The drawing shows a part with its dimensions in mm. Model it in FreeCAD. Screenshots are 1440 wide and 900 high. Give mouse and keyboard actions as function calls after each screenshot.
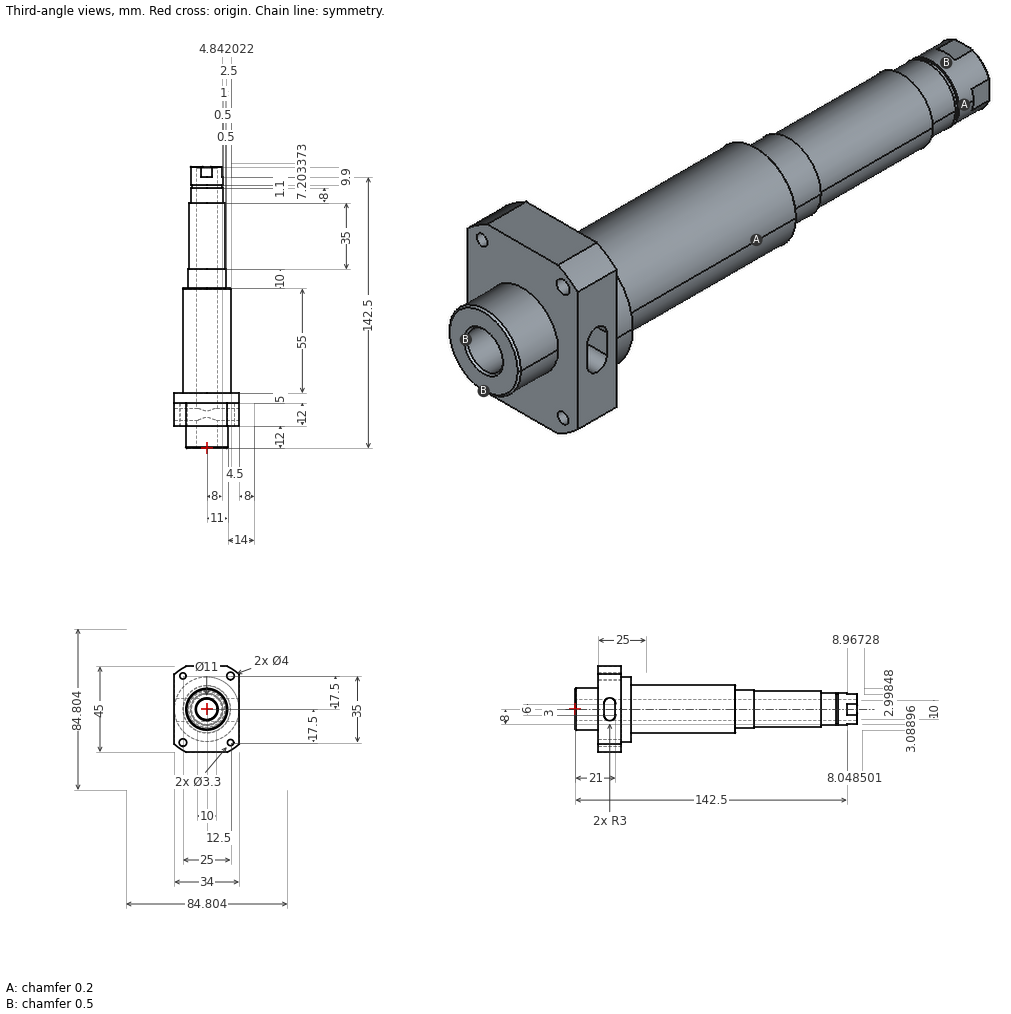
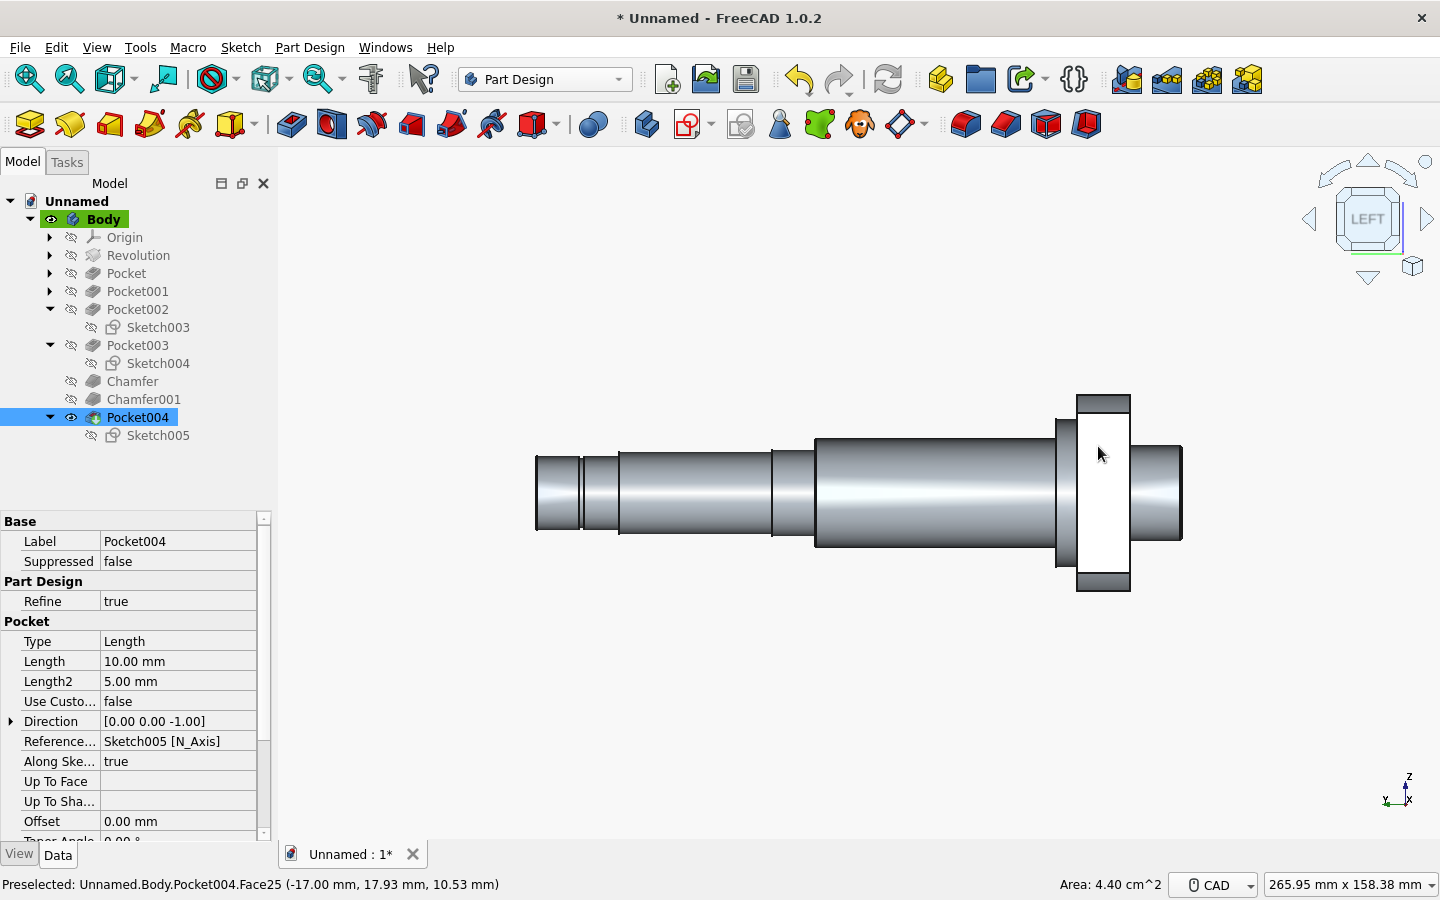
click(688, 124)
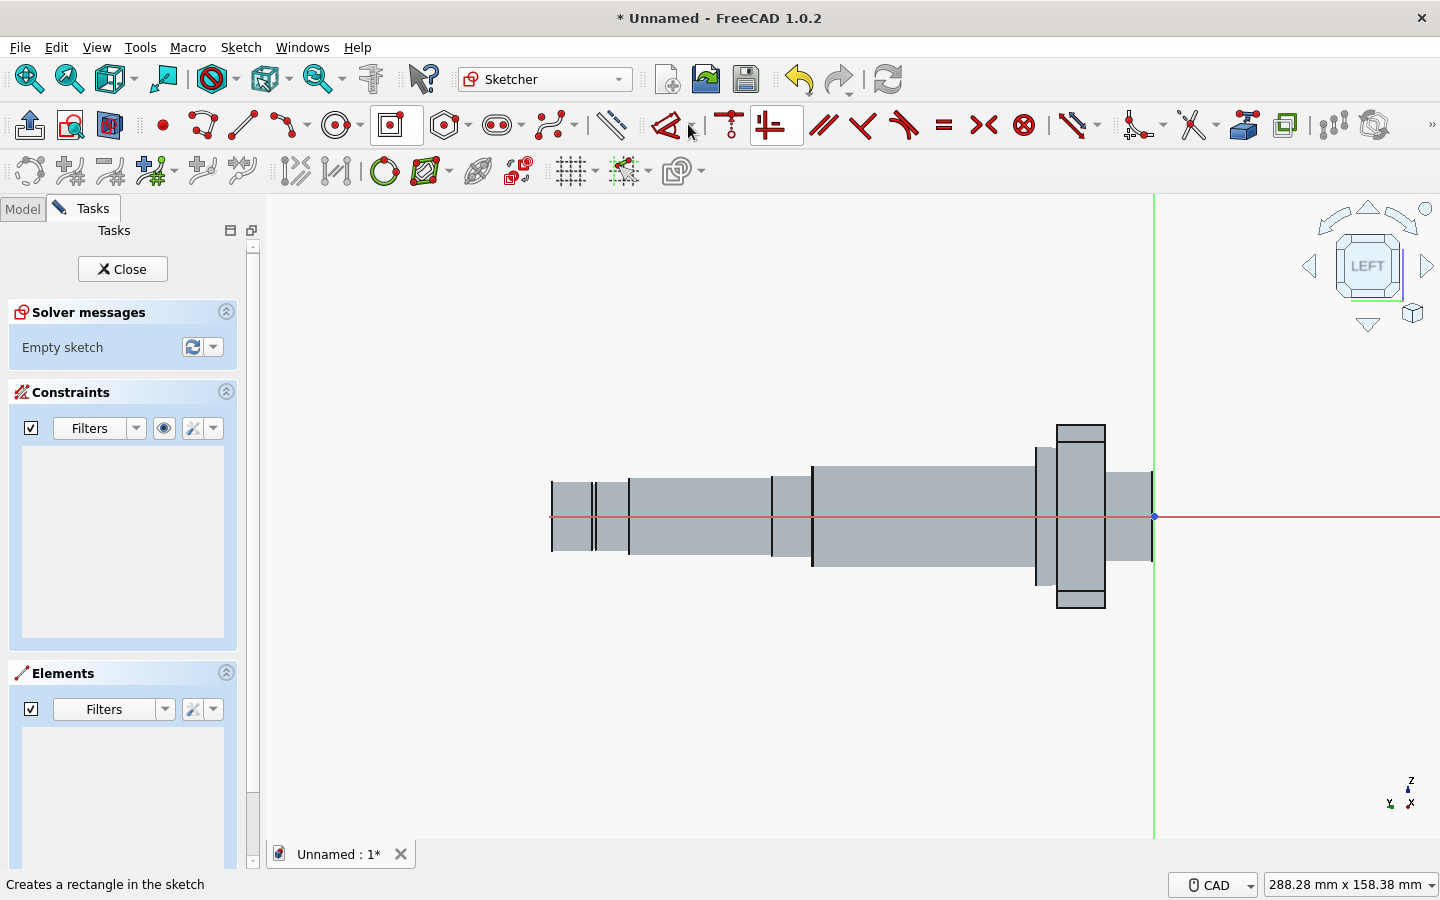
scroll(1163, 516, up, 10)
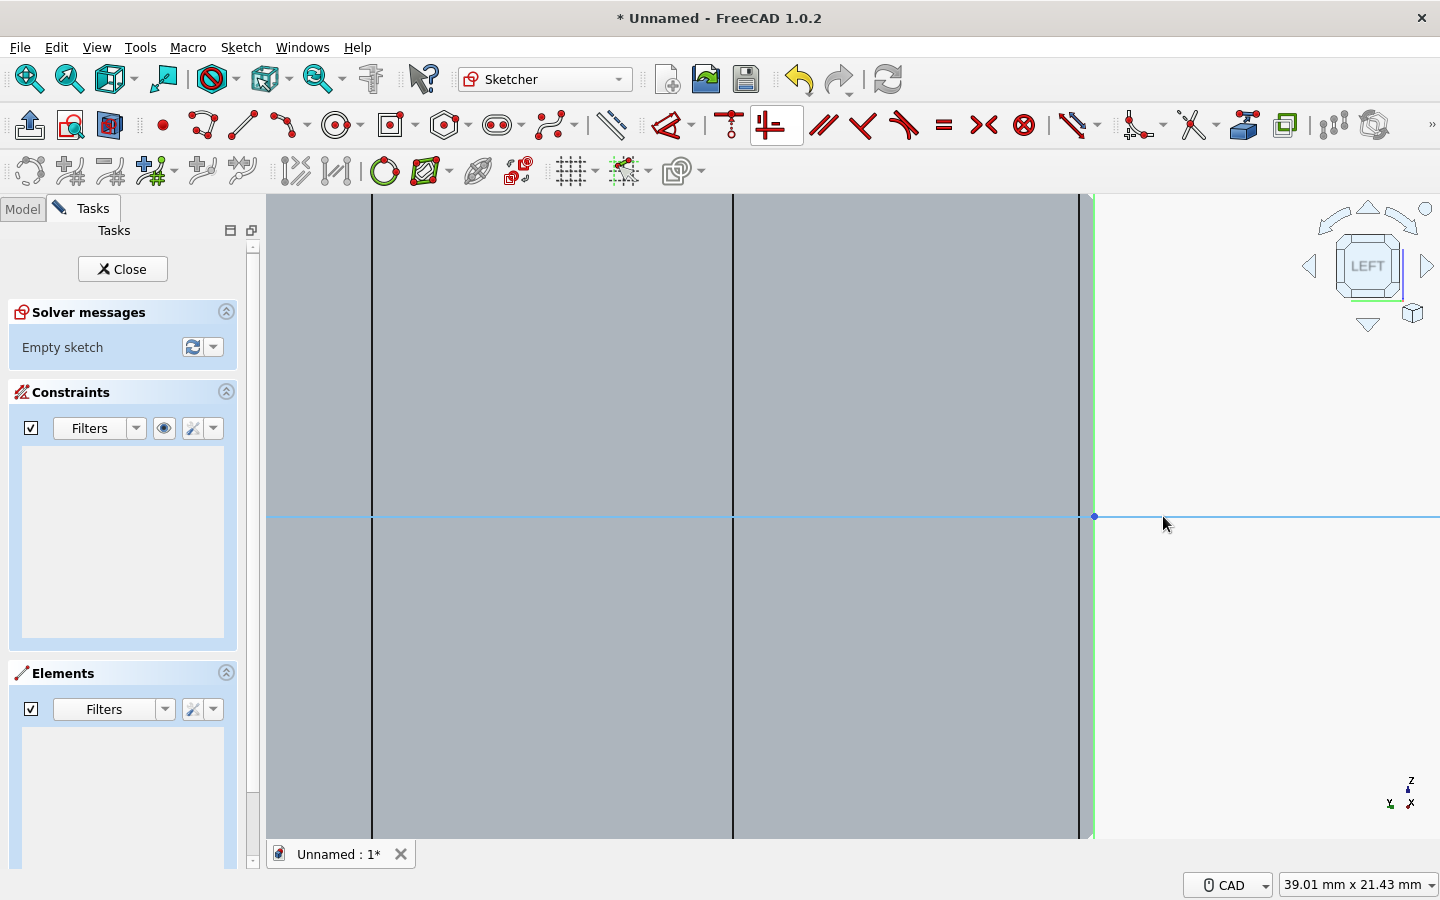
key(g)
key(s)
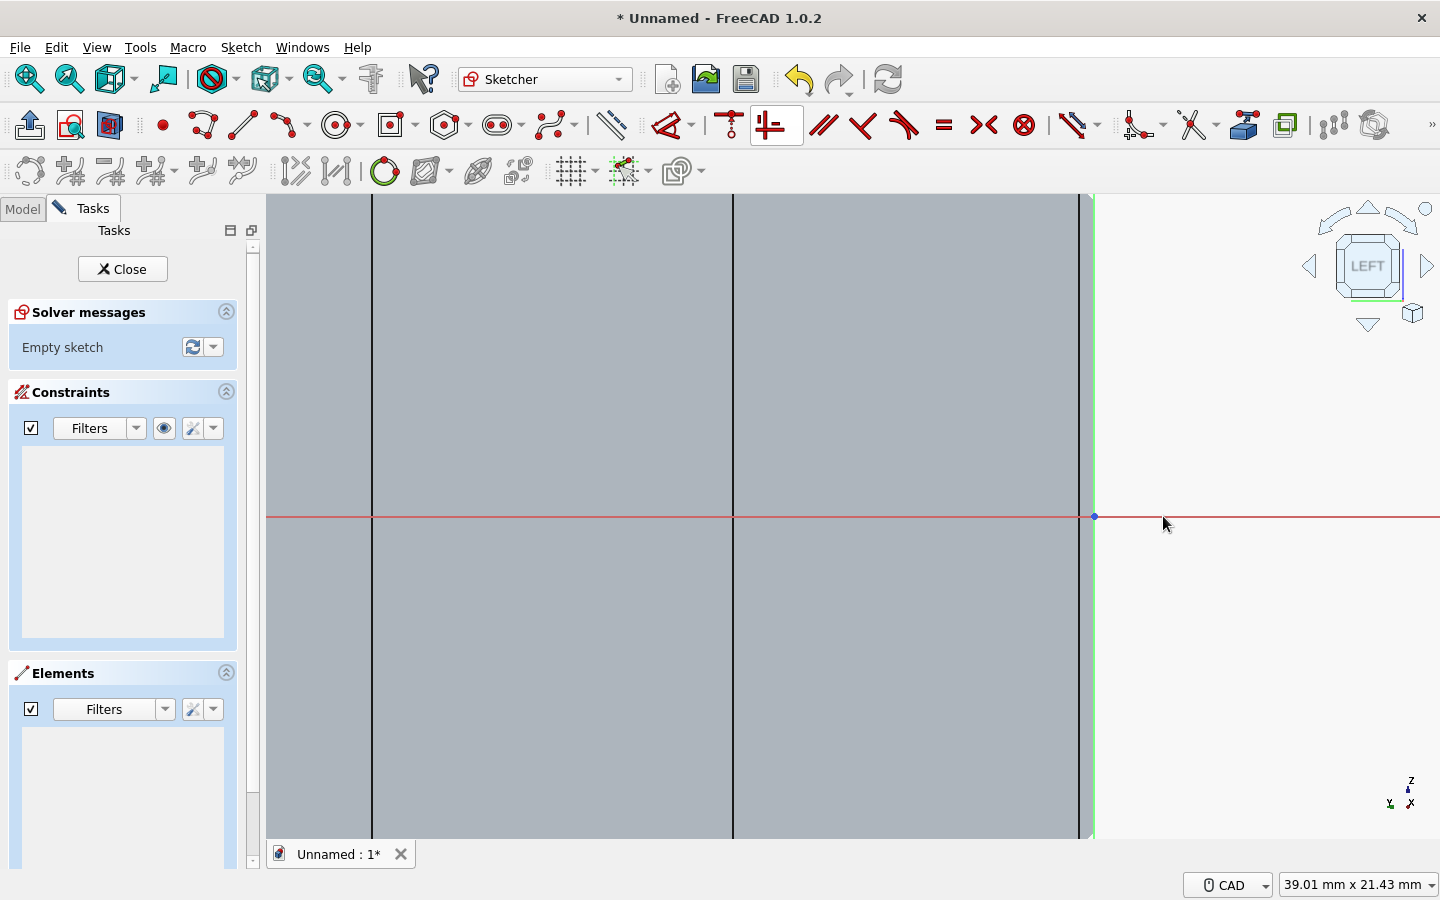
click(553, 607)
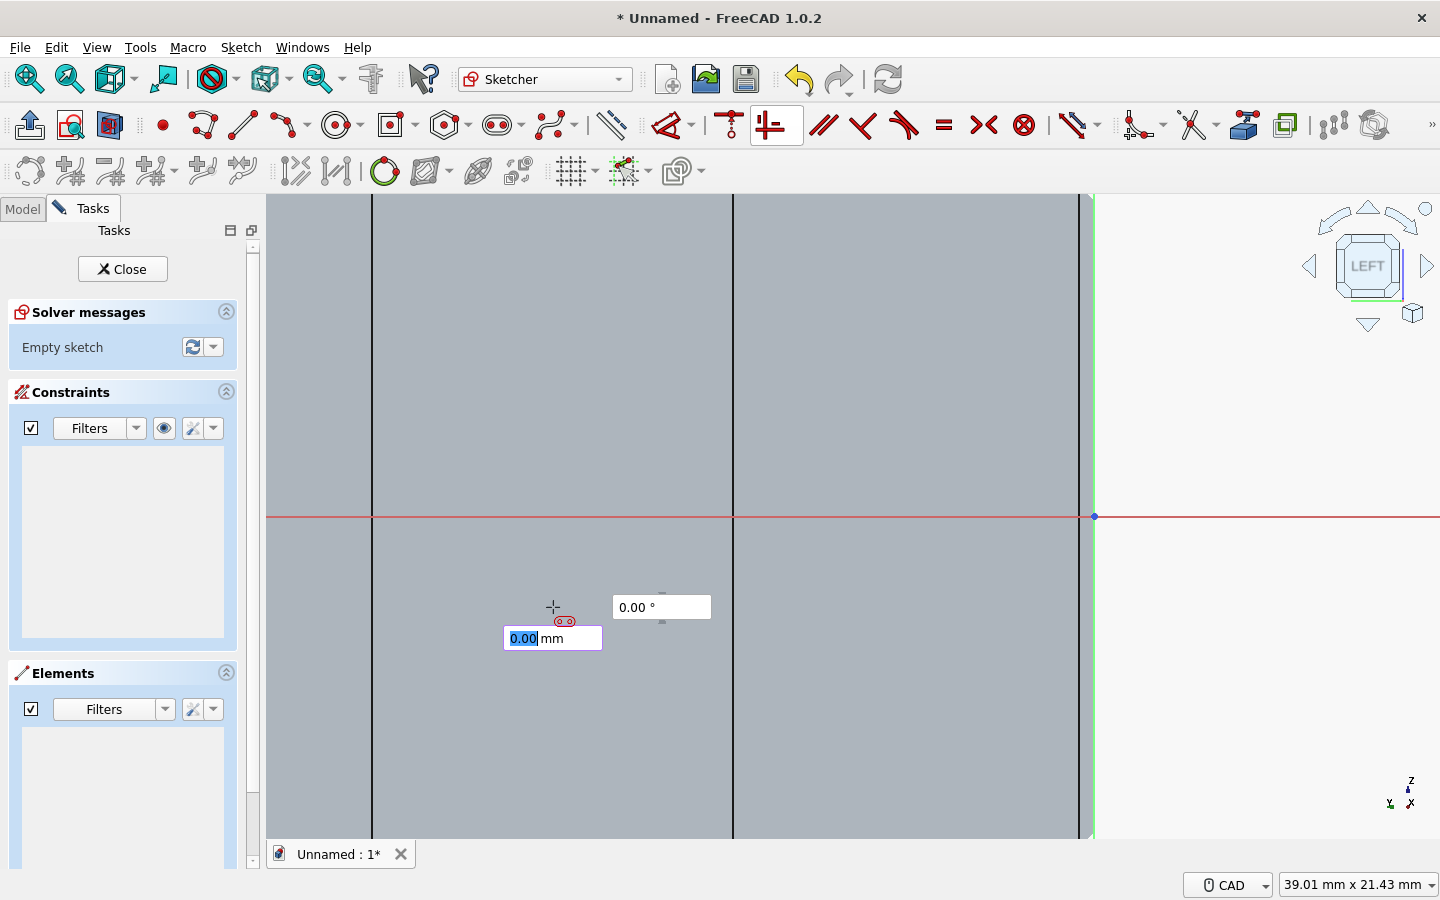
click(553, 426)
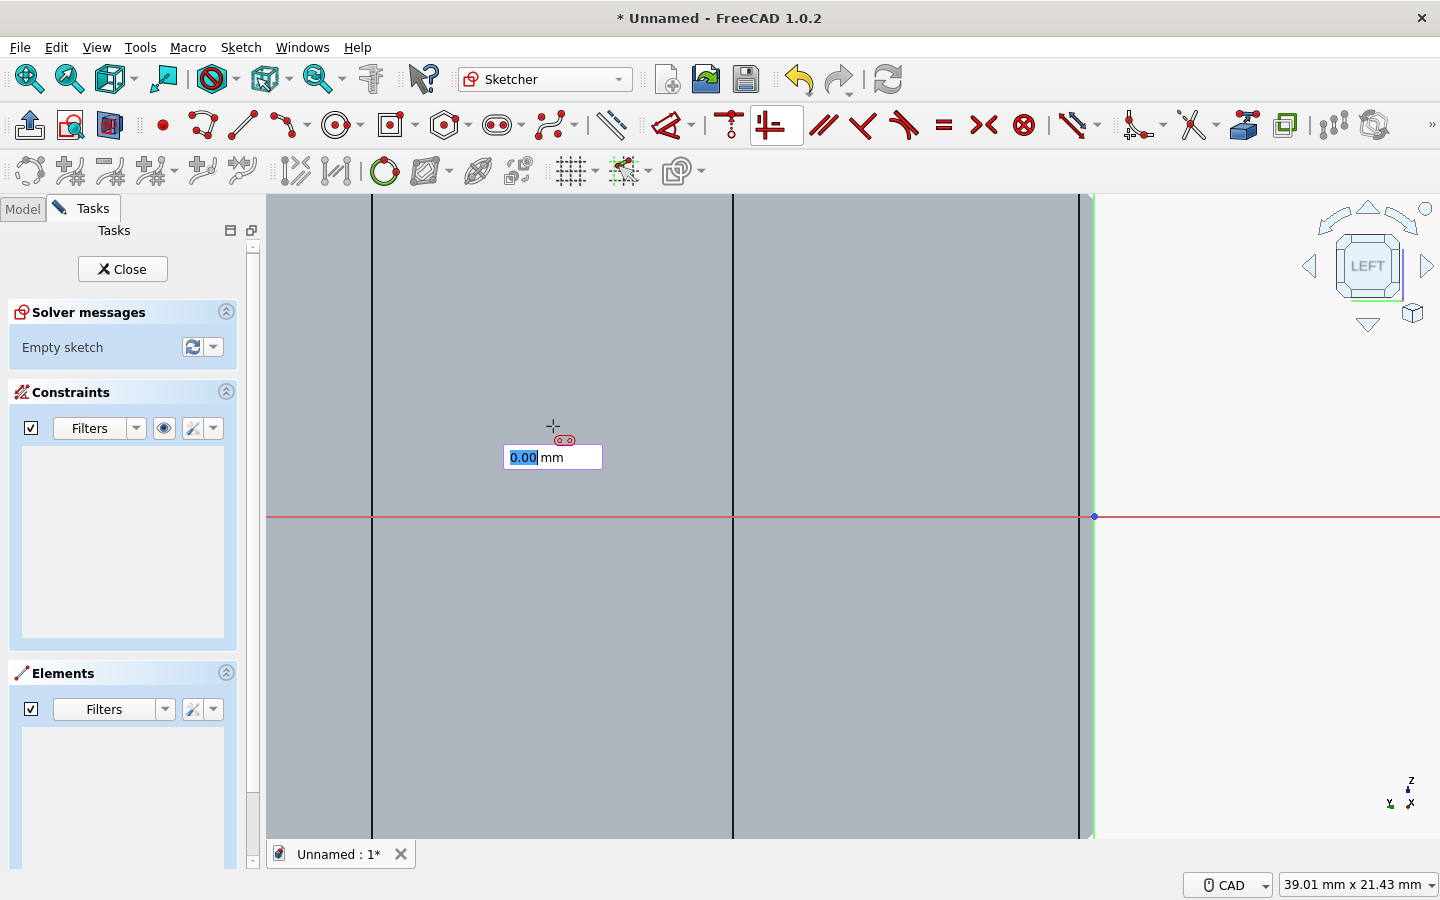
click(462, 489)
key(Escape)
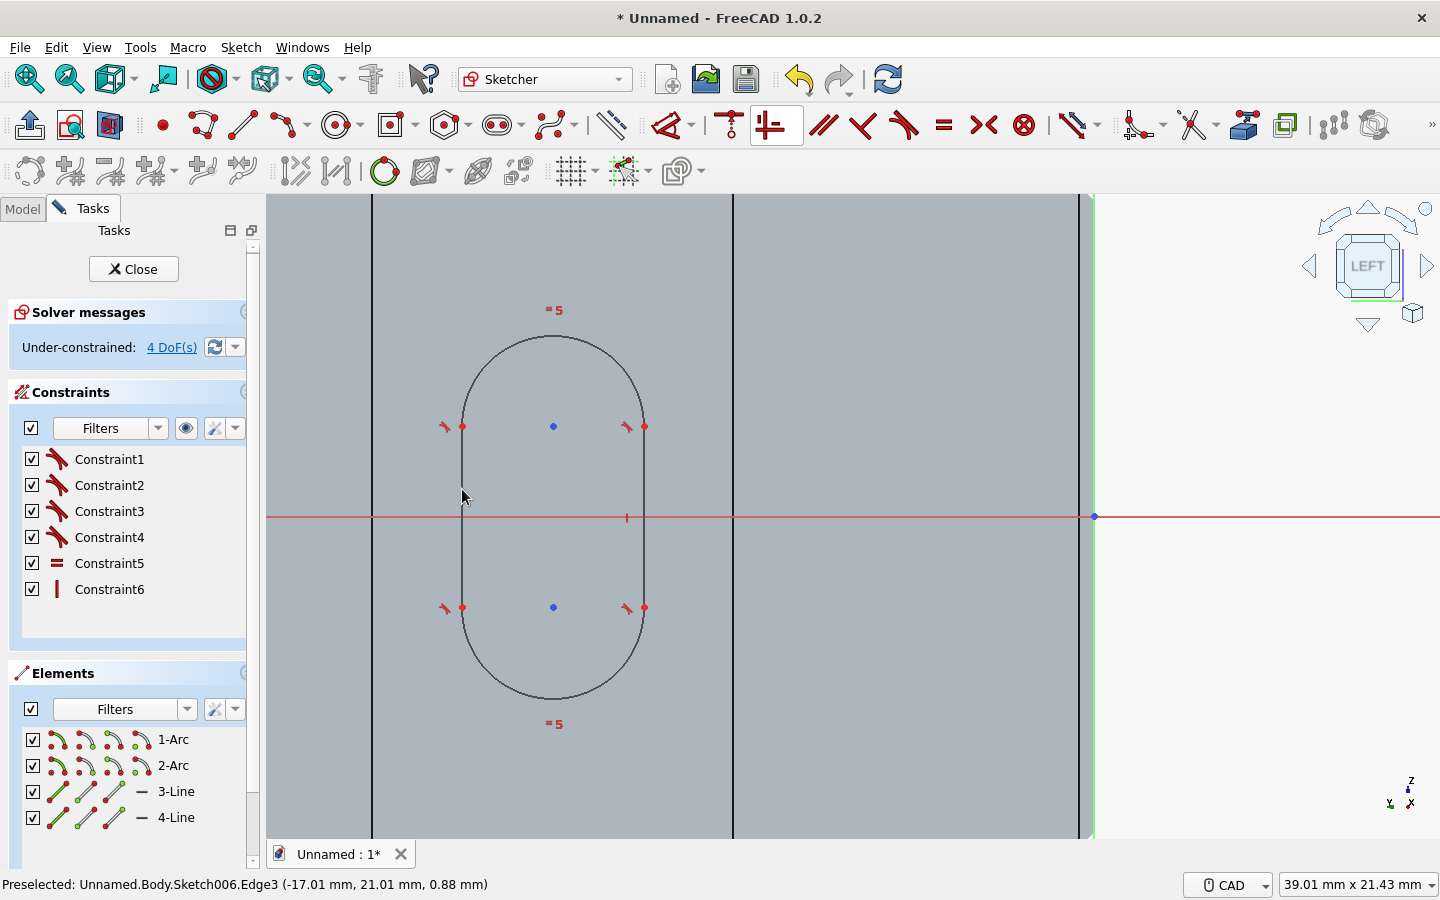
key(d)